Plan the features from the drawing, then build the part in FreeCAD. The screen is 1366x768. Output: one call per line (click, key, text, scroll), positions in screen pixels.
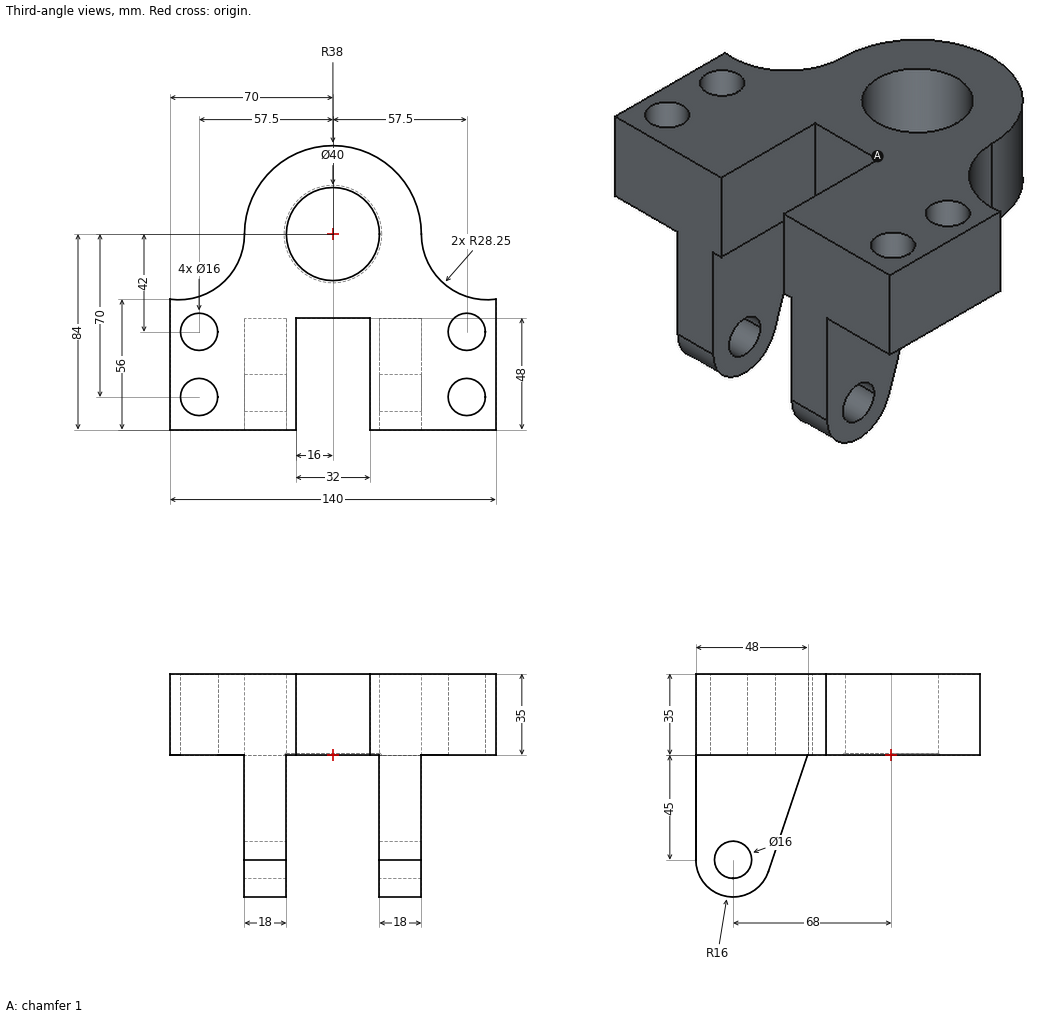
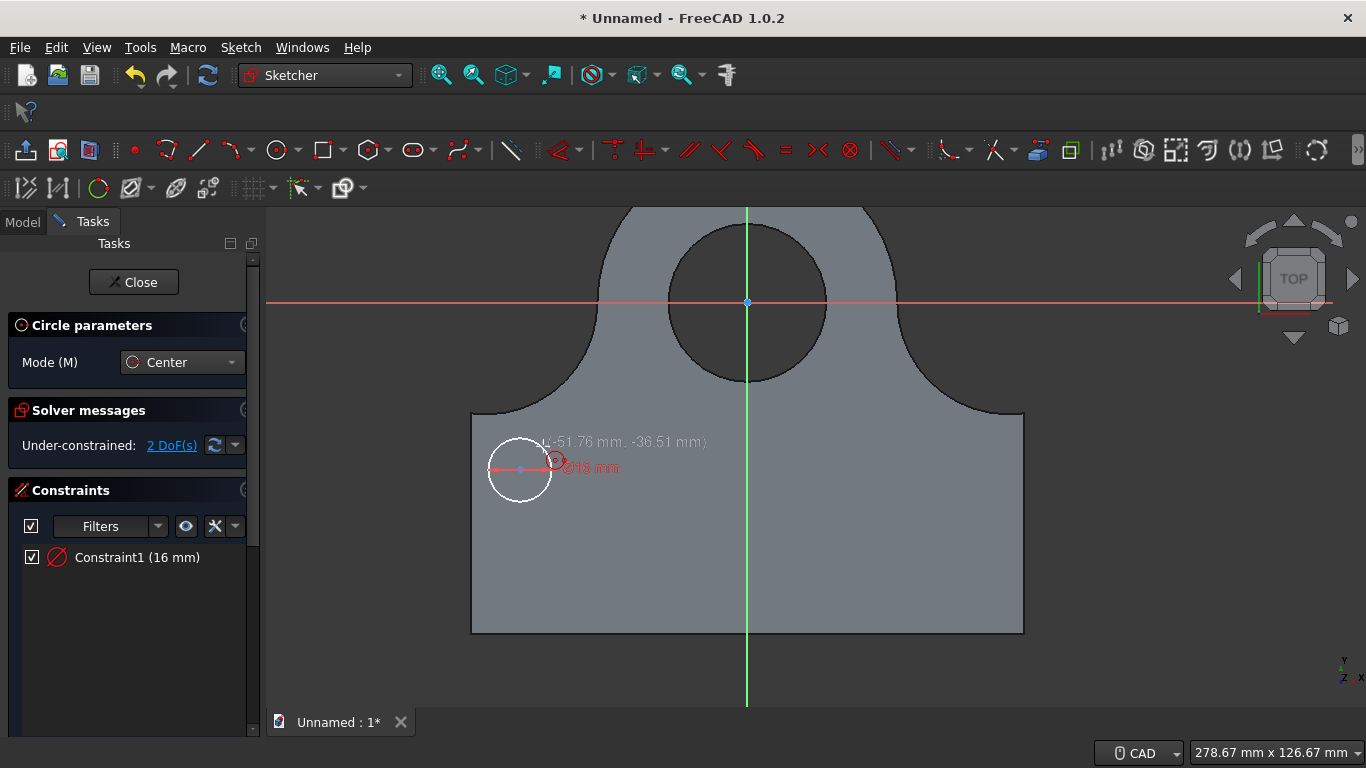
click(520, 579)
move(543, 557)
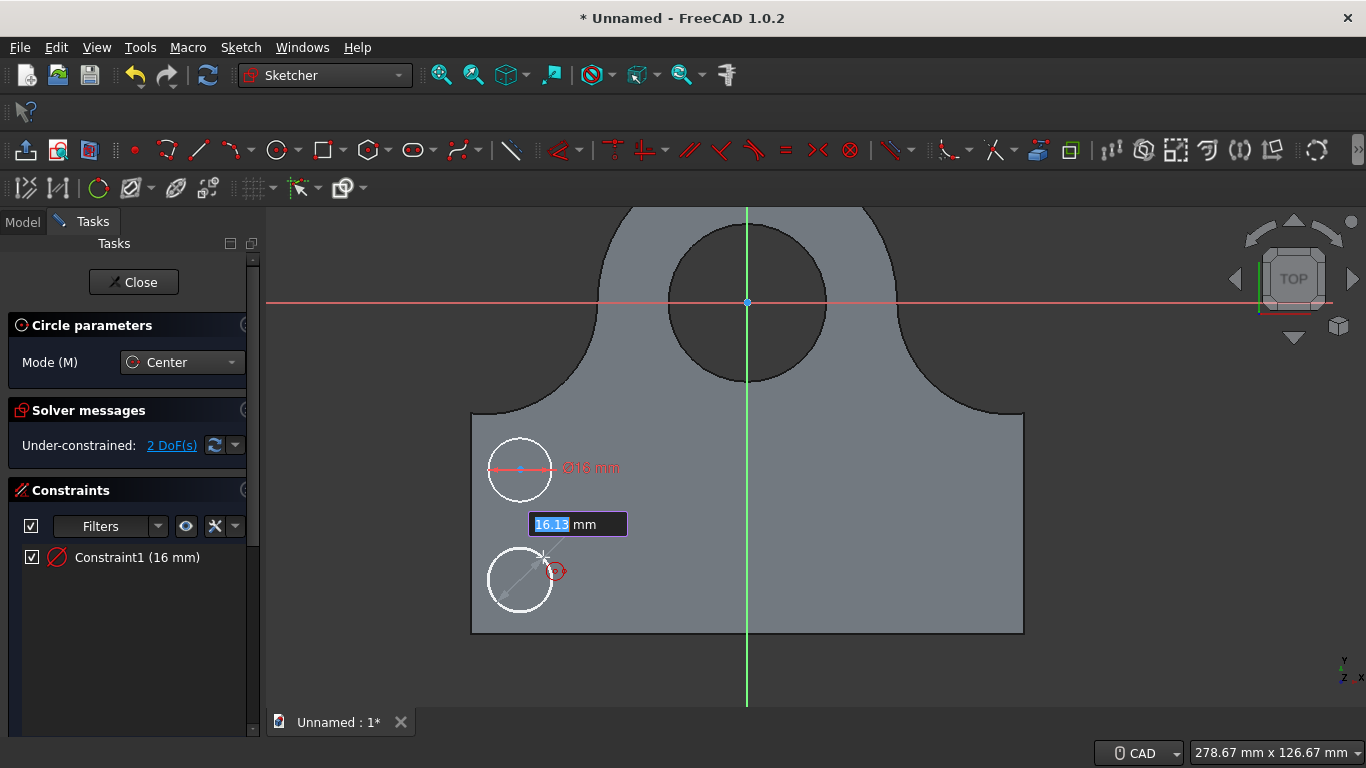
text(16)
key(Return)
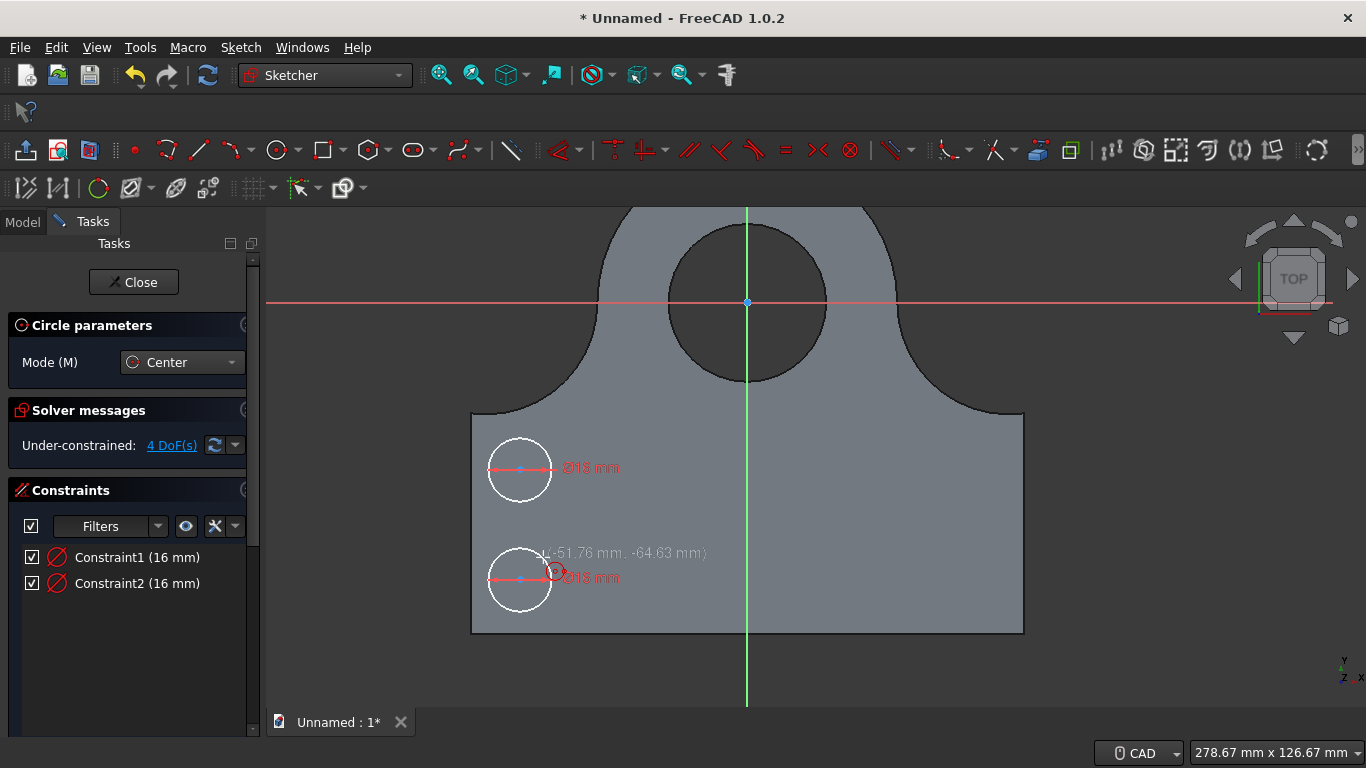
click(974, 469)
move(997, 446)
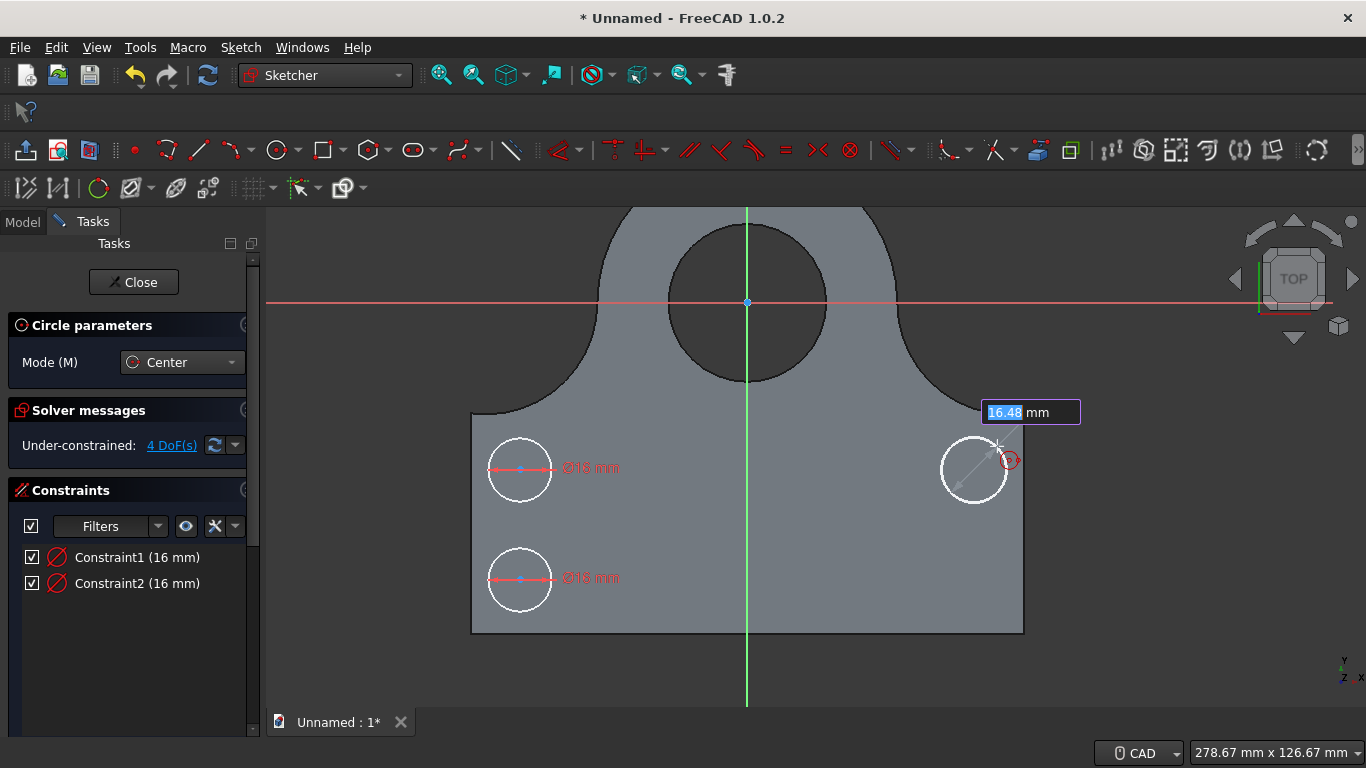
text(16)
key(Return)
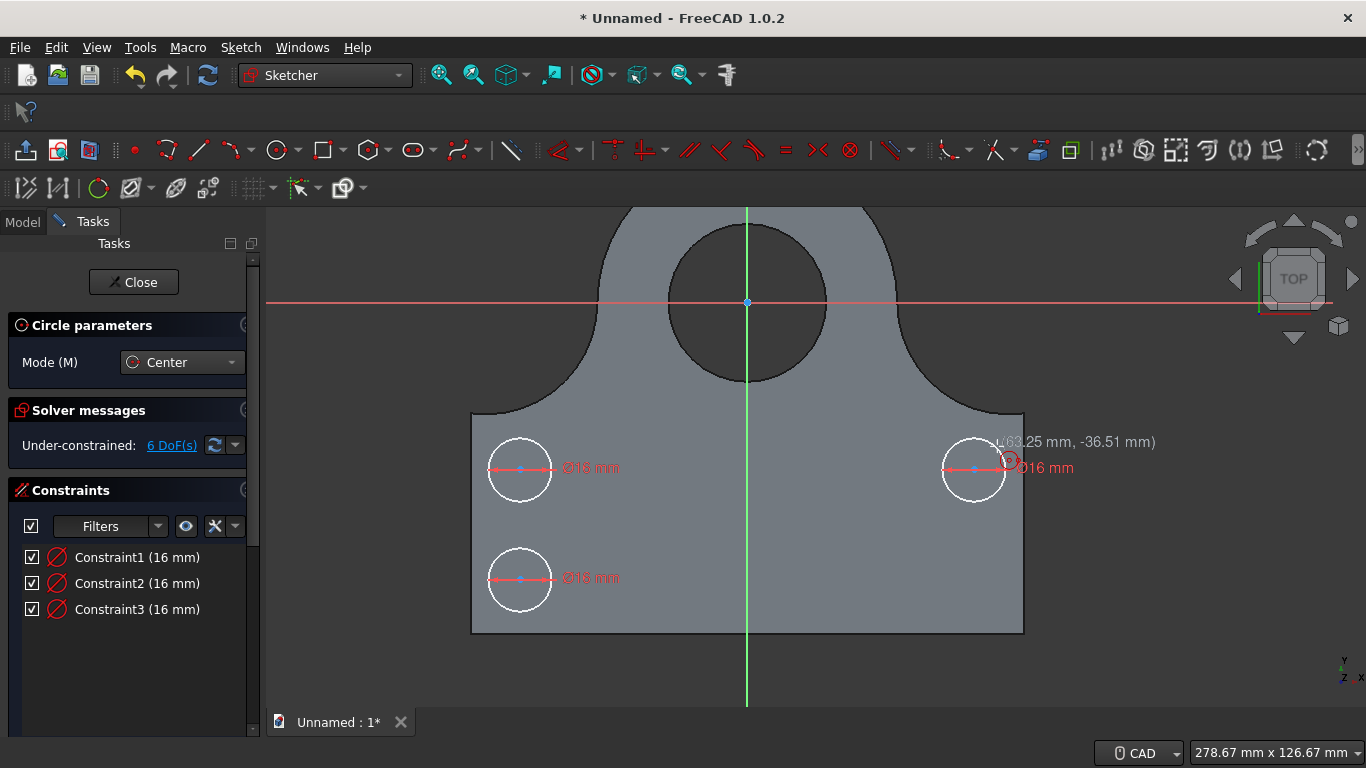
click(974, 579)
move(997, 557)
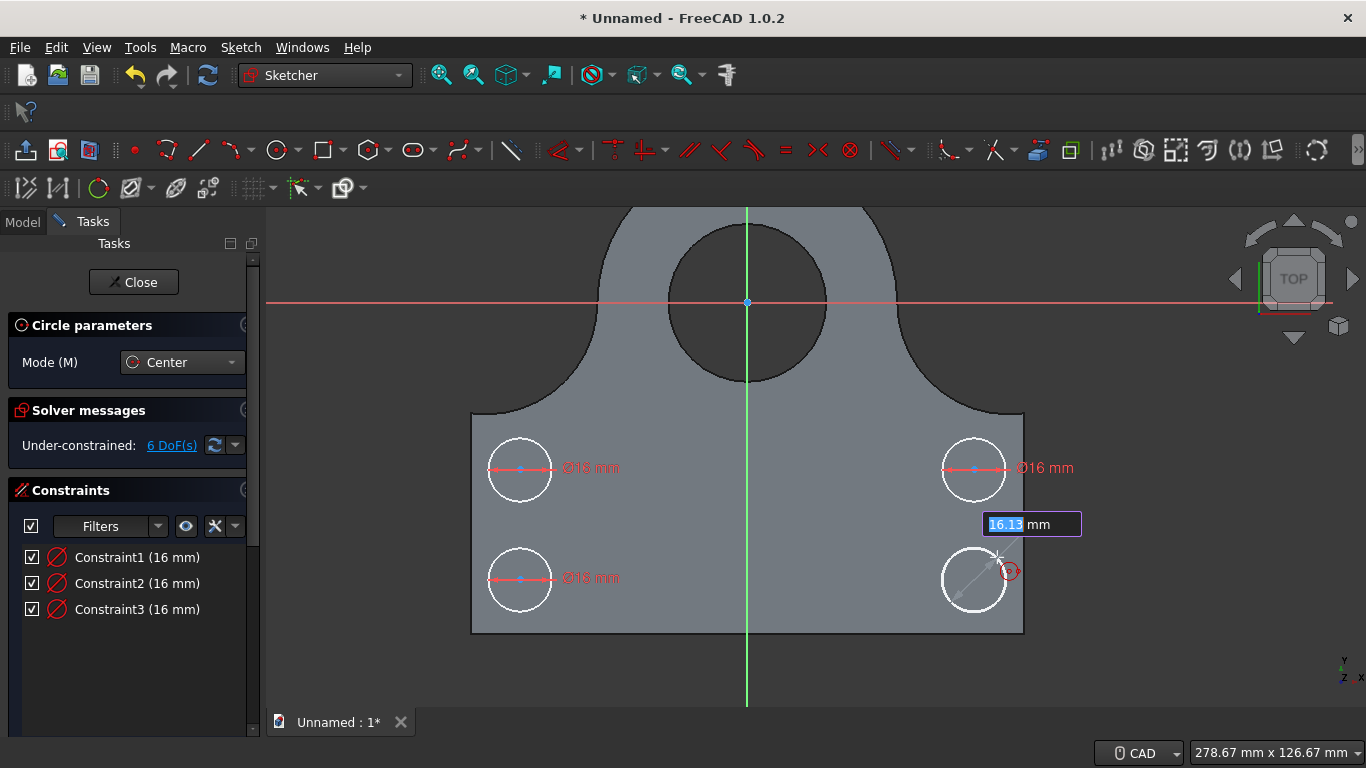
text(16)
key(Return)
key(Escape)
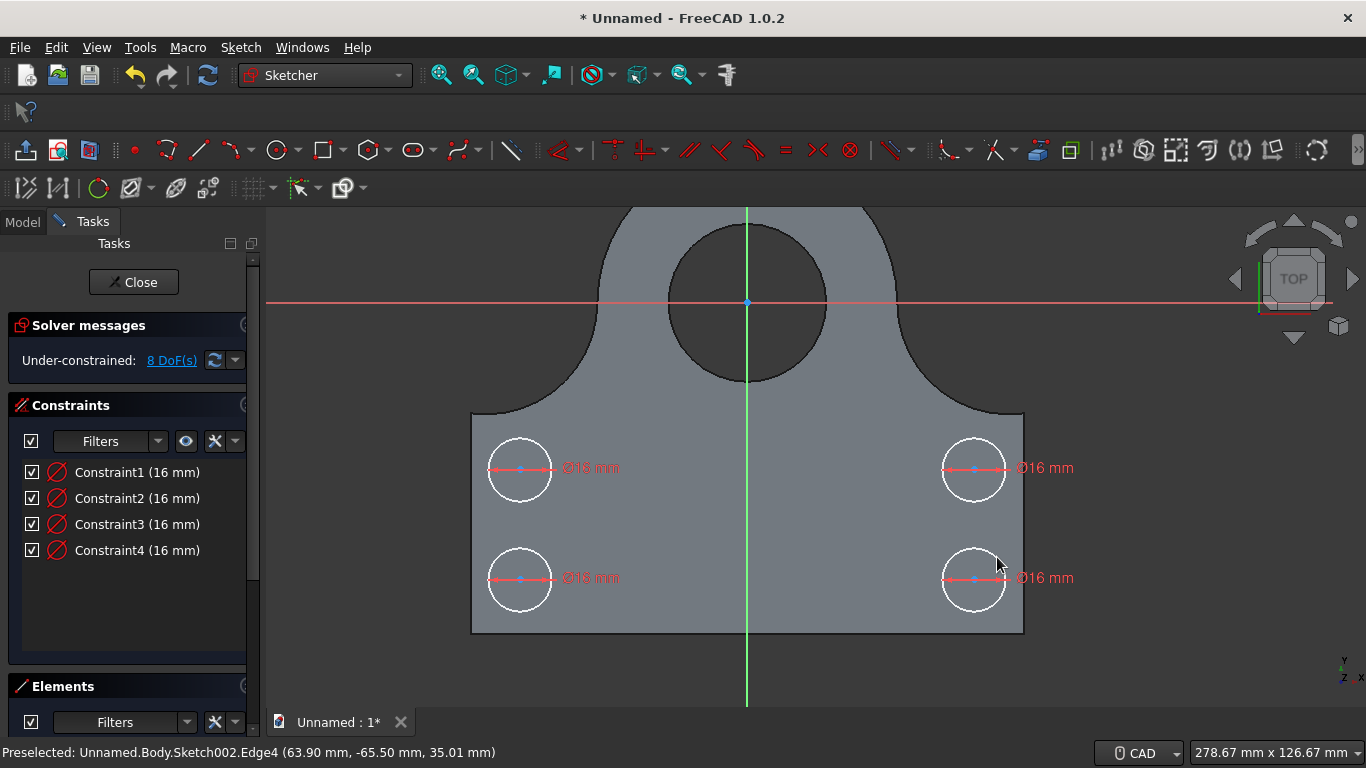
click(520, 470)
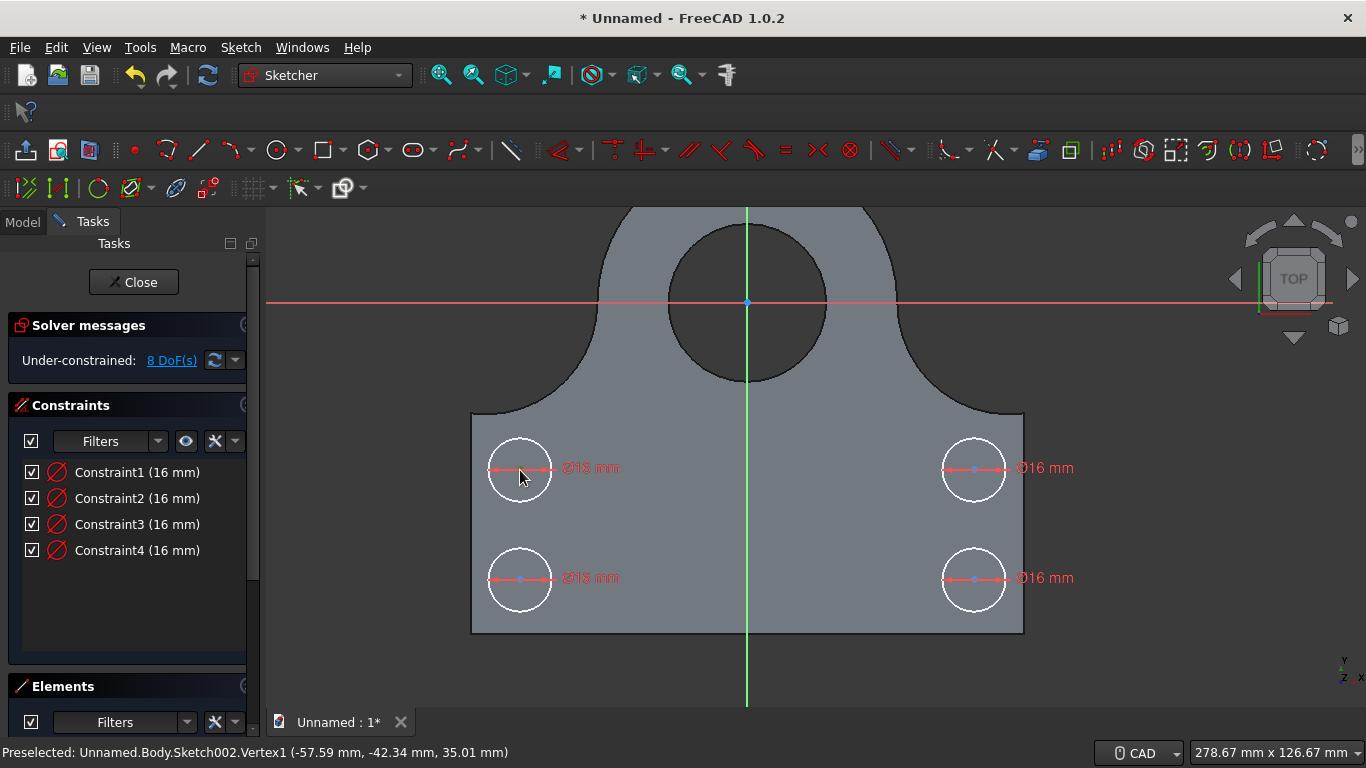
click(520, 580)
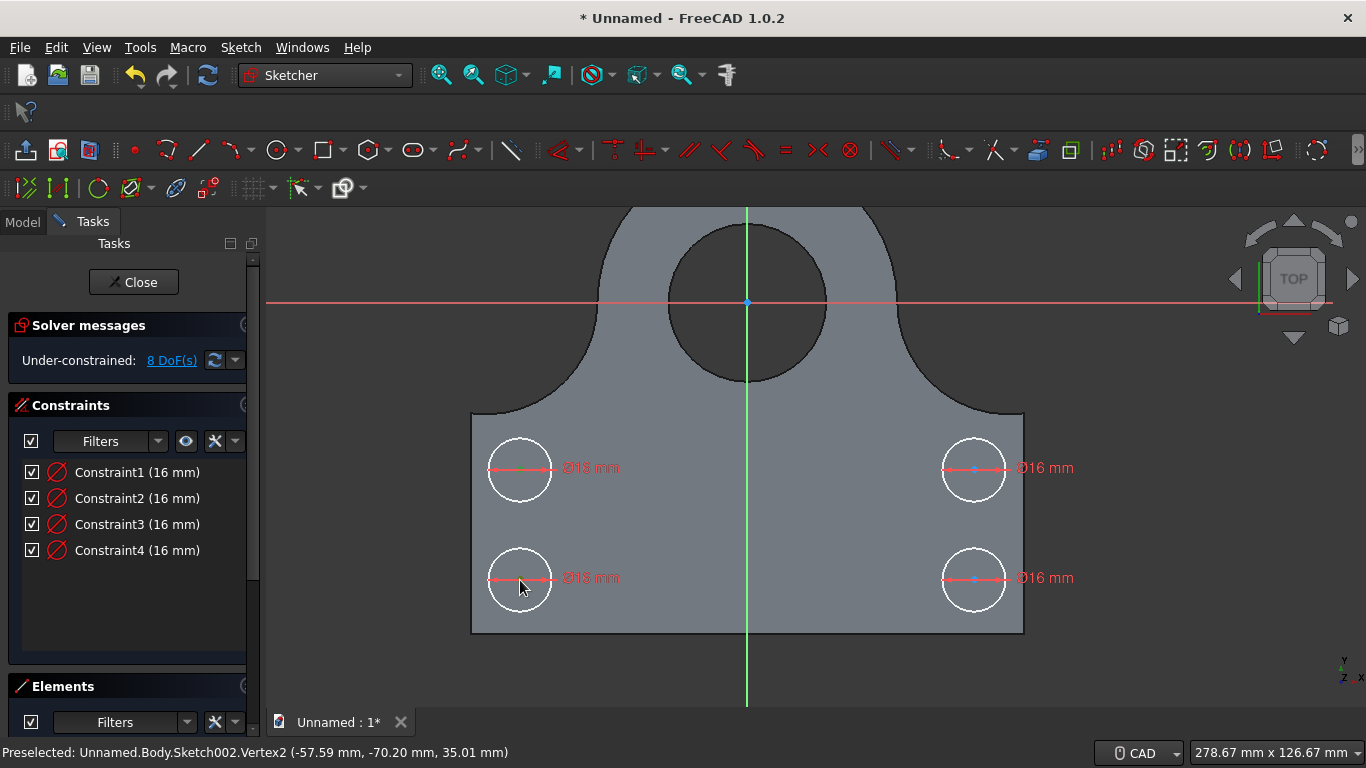
key(v)